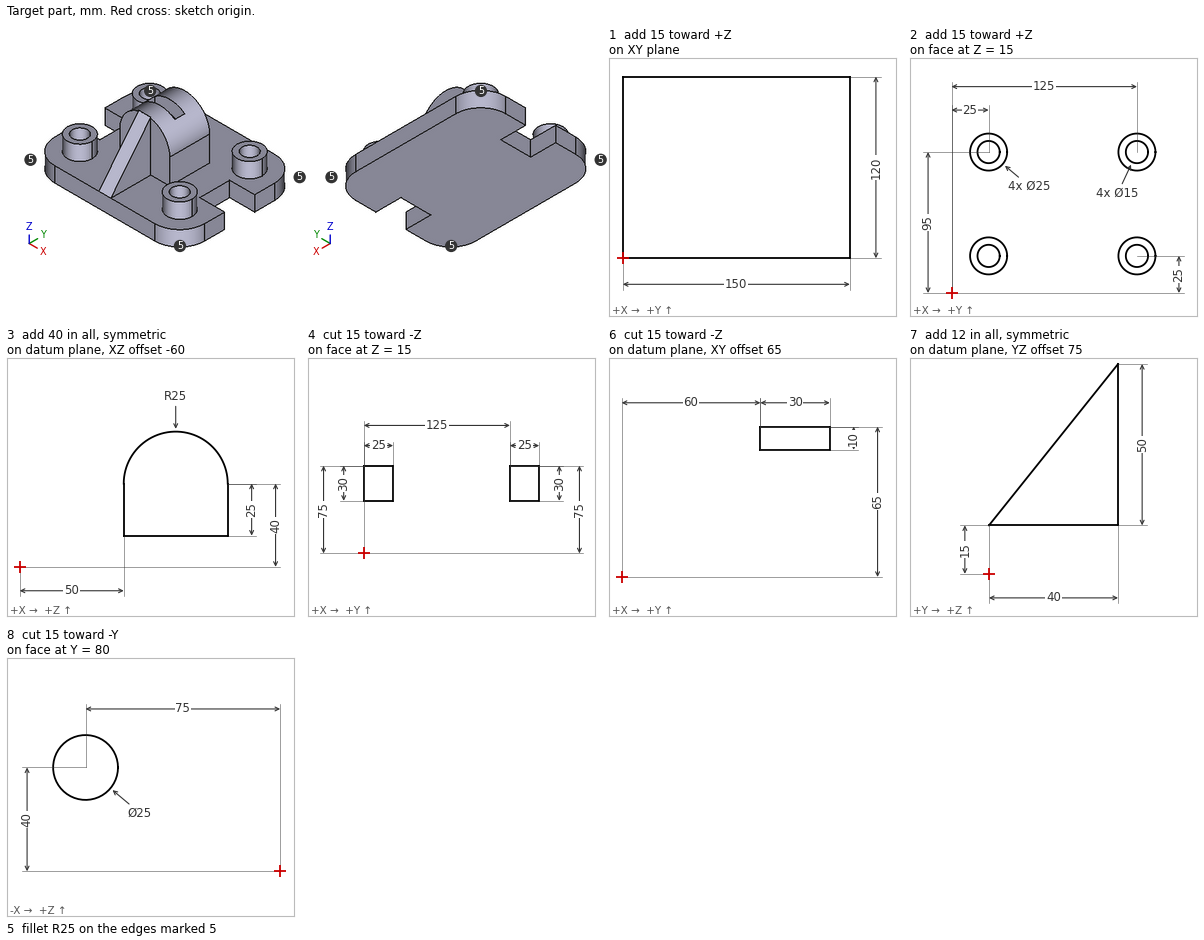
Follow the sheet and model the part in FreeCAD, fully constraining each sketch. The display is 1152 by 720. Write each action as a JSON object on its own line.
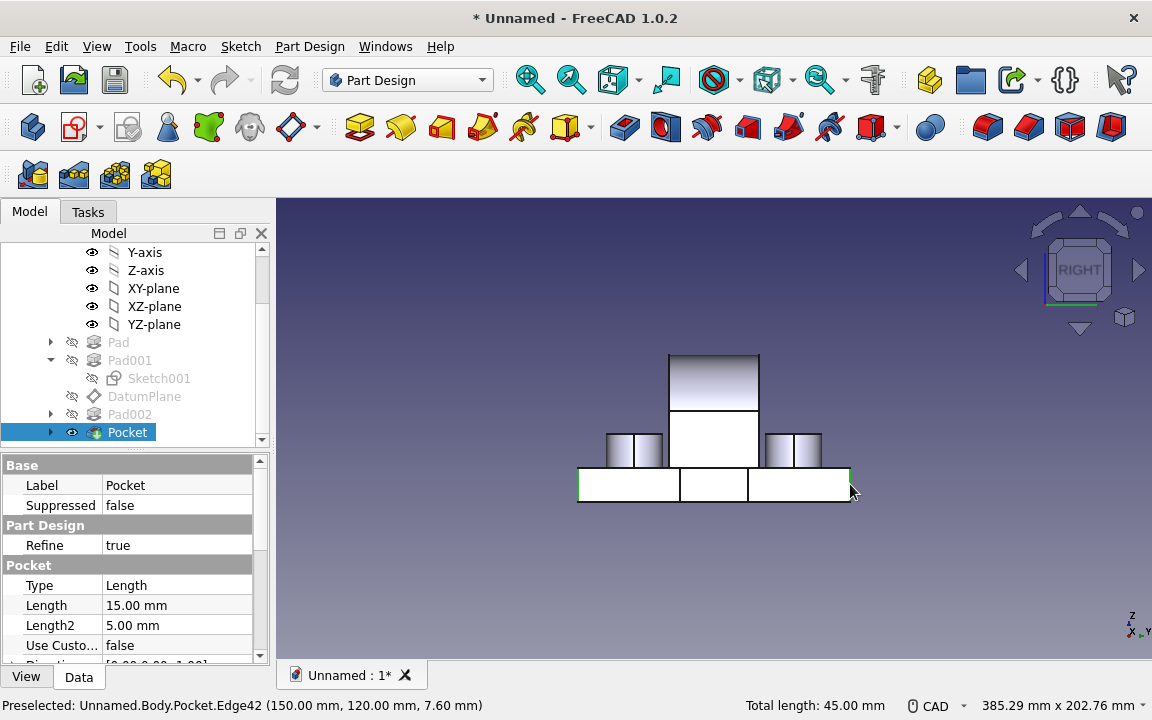
{"action": "key", "text": "5"}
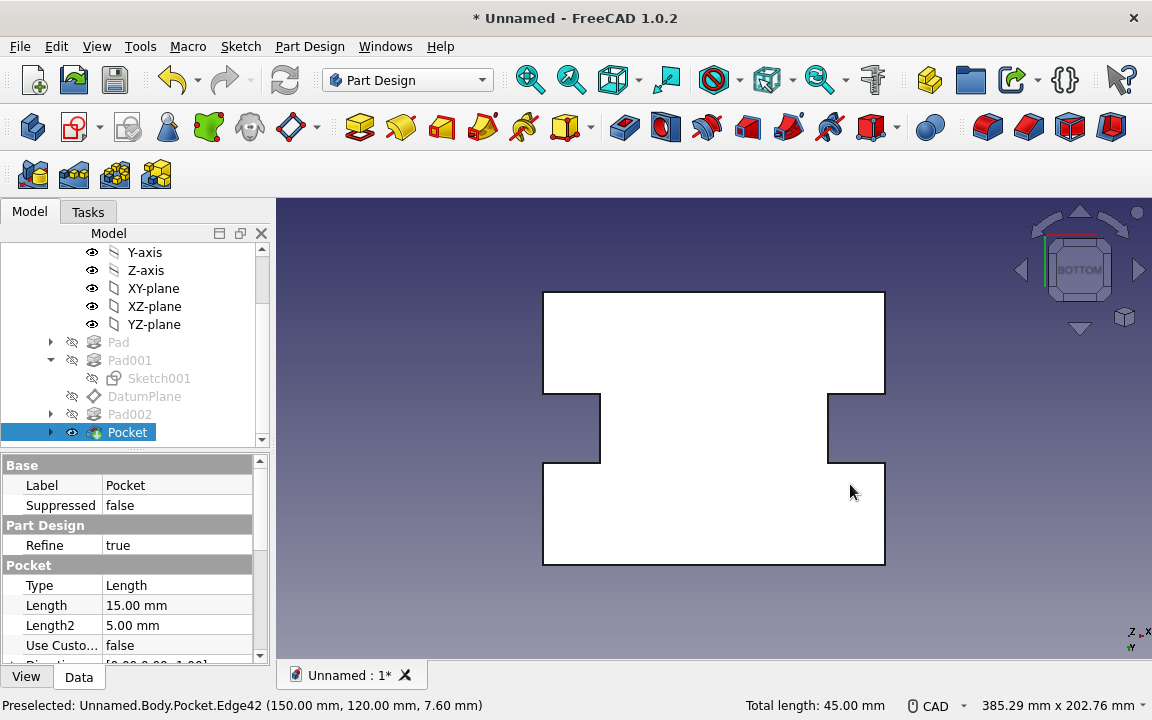
{"action": "key", "text": "4"}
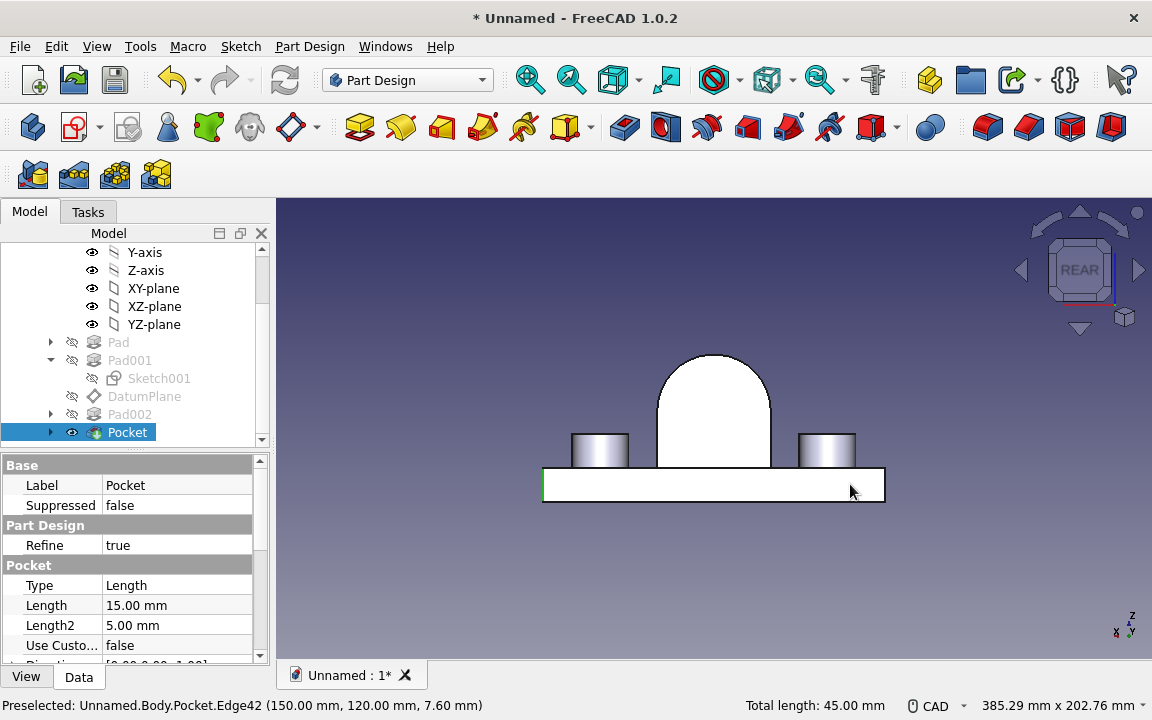
{"action": "left_click", "coordinate": [531, 80]}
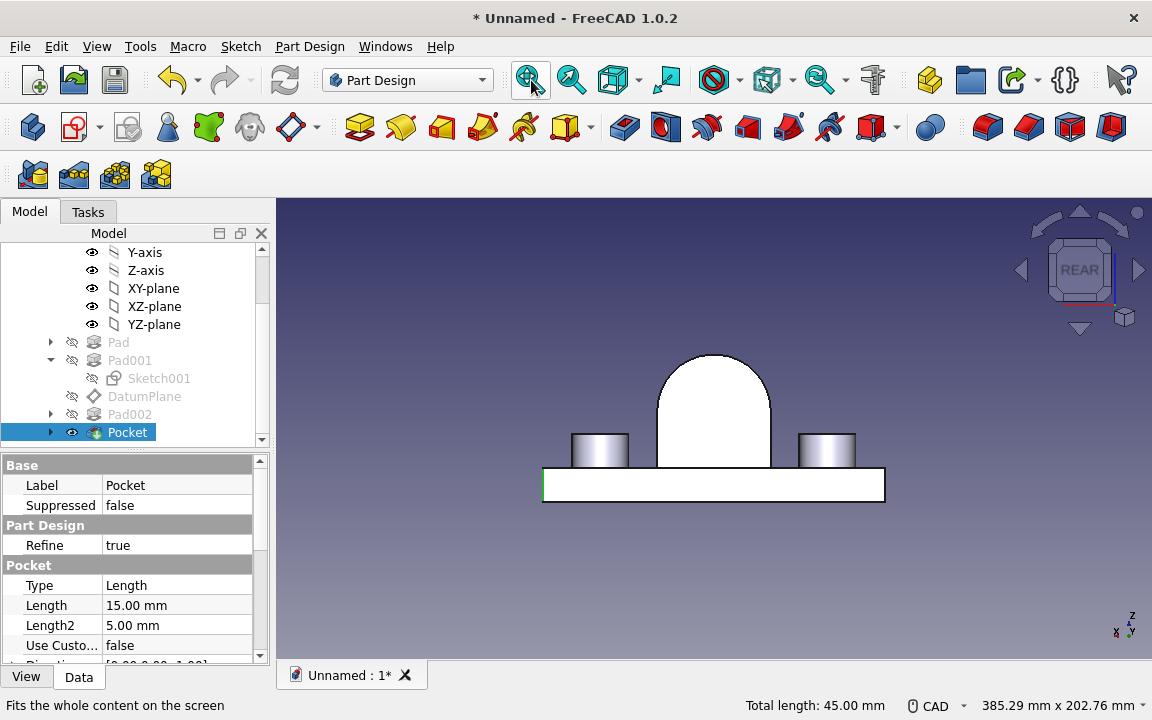
{"action": "left_click", "coordinate": [885, 484], "text": "ctrl"}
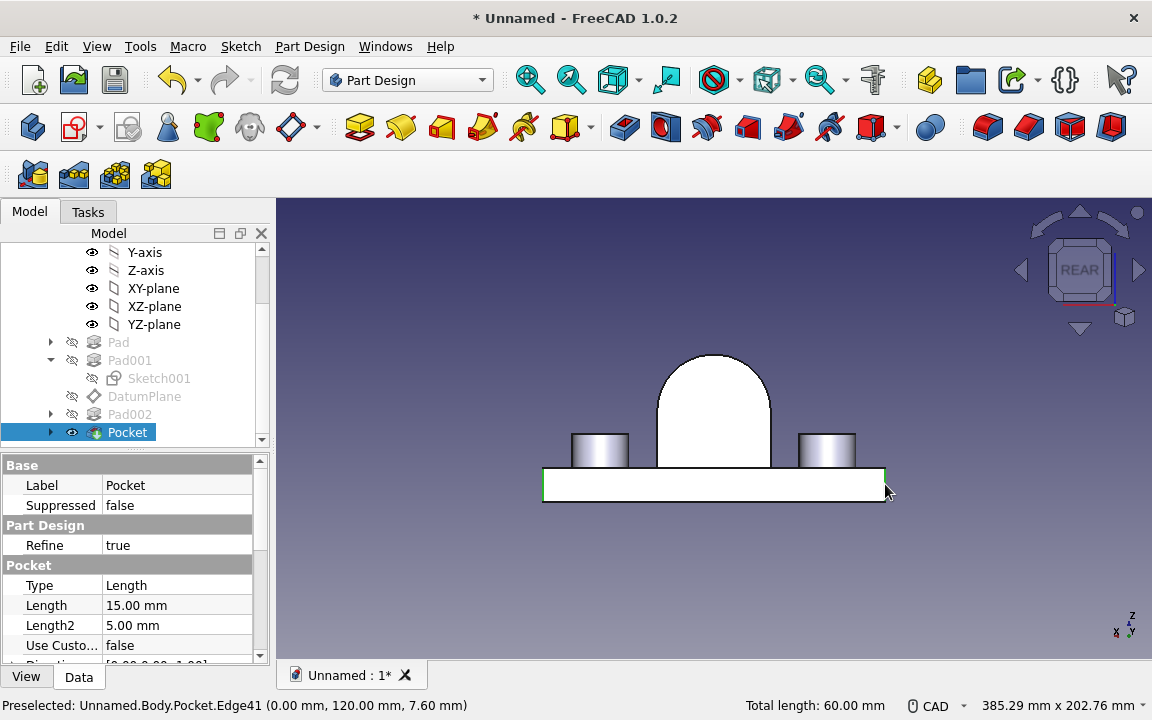
{"action": "left_click", "coordinate": [988, 128]}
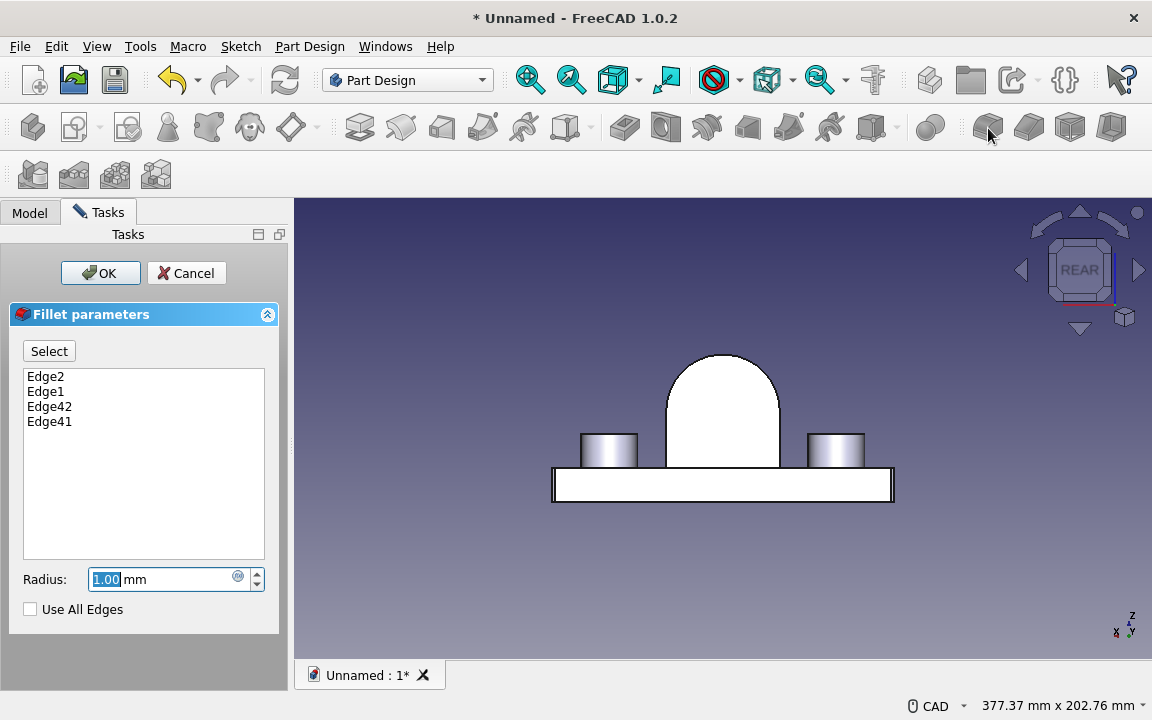
{"action": "type", "text": "25"}
{"action": "key", "text": "Tab"}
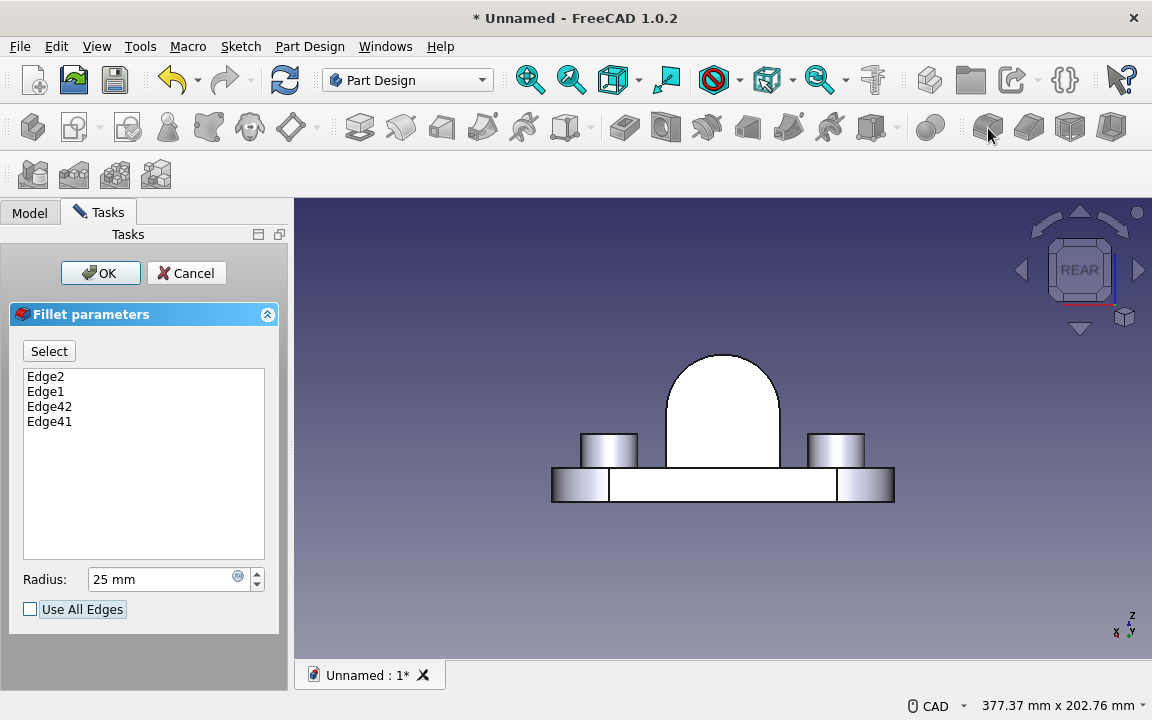
{"action": "left_click", "coordinate": [101, 273]}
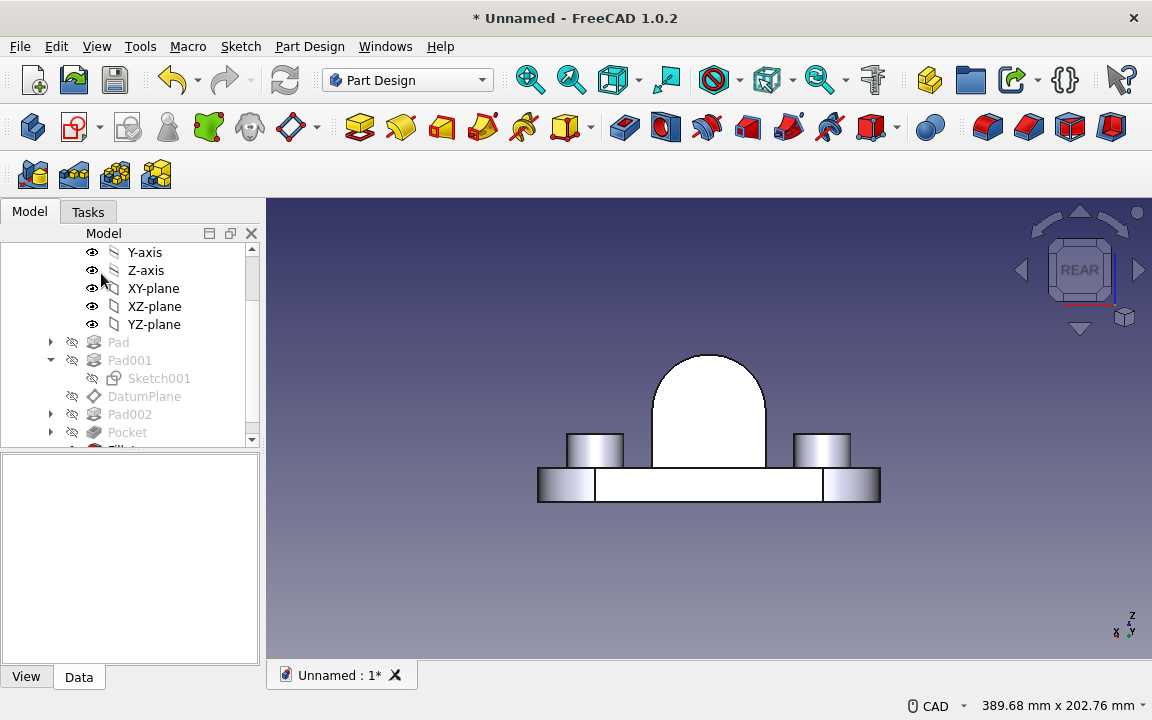
{"action": "left_click", "coordinate": [531, 80]}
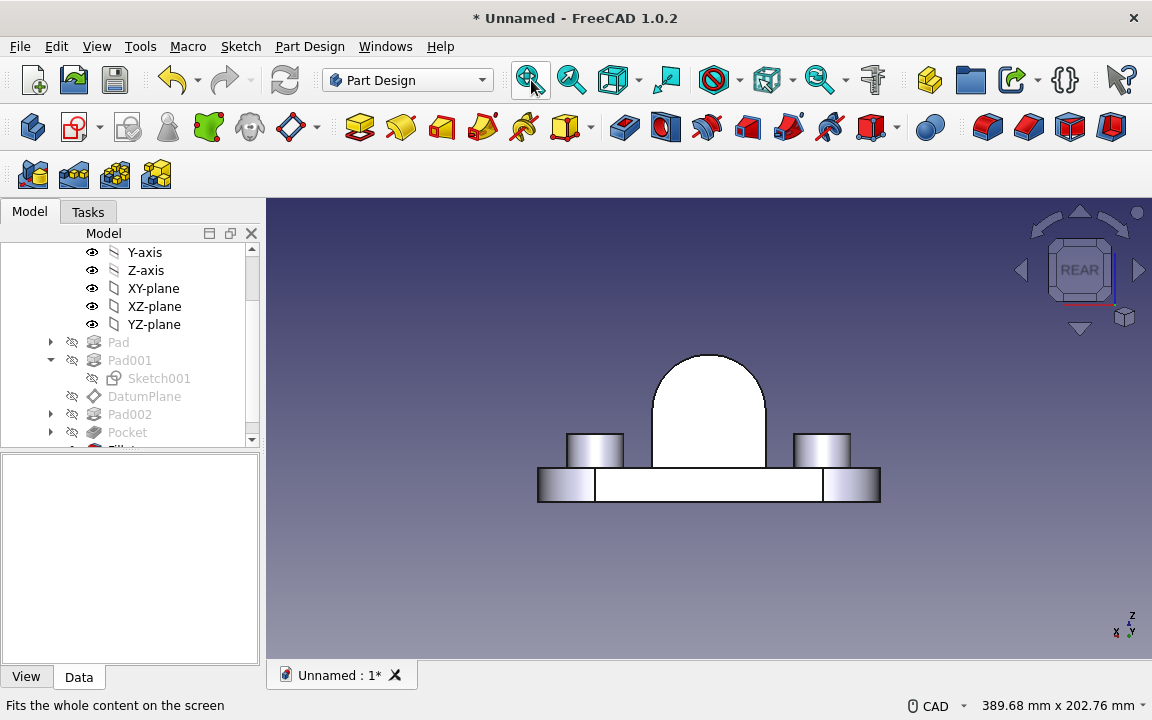
{"action": "scroll", "coordinate": [161, 338], "scroll_direction": "down", "scroll_amount": 3}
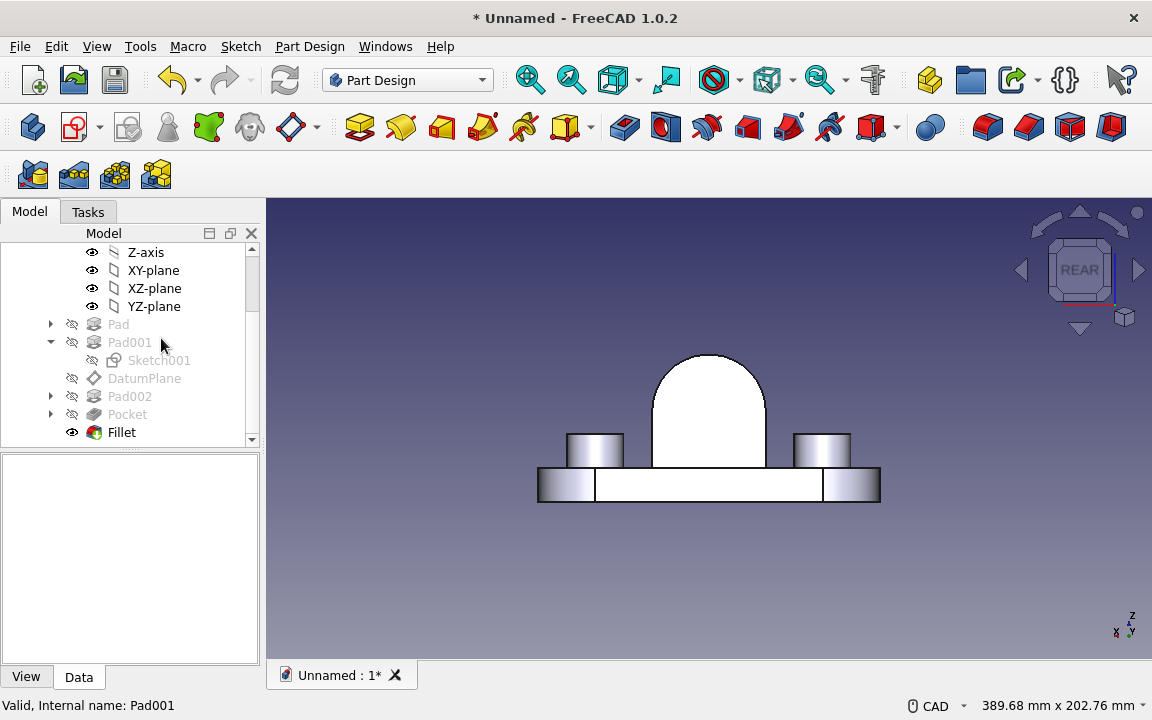
{"action": "scroll", "coordinate": [161, 338], "scroll_direction": "up", "scroll_amount": 15}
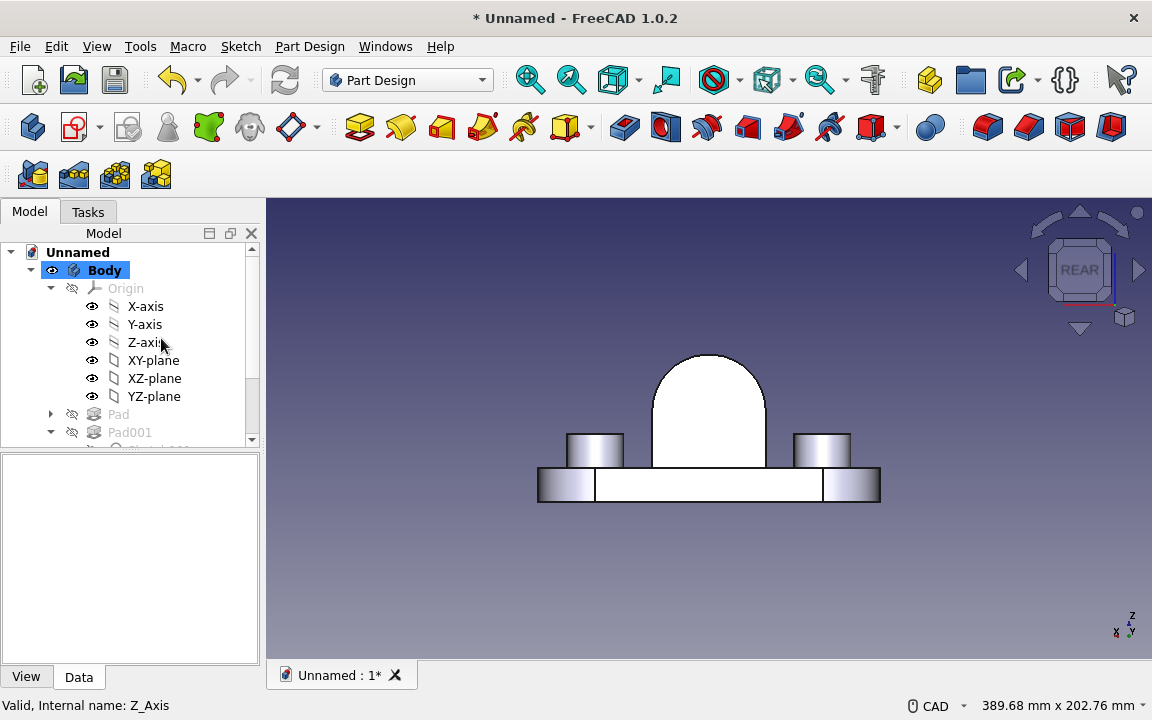
{"action": "left_click", "coordinate": [137, 360]}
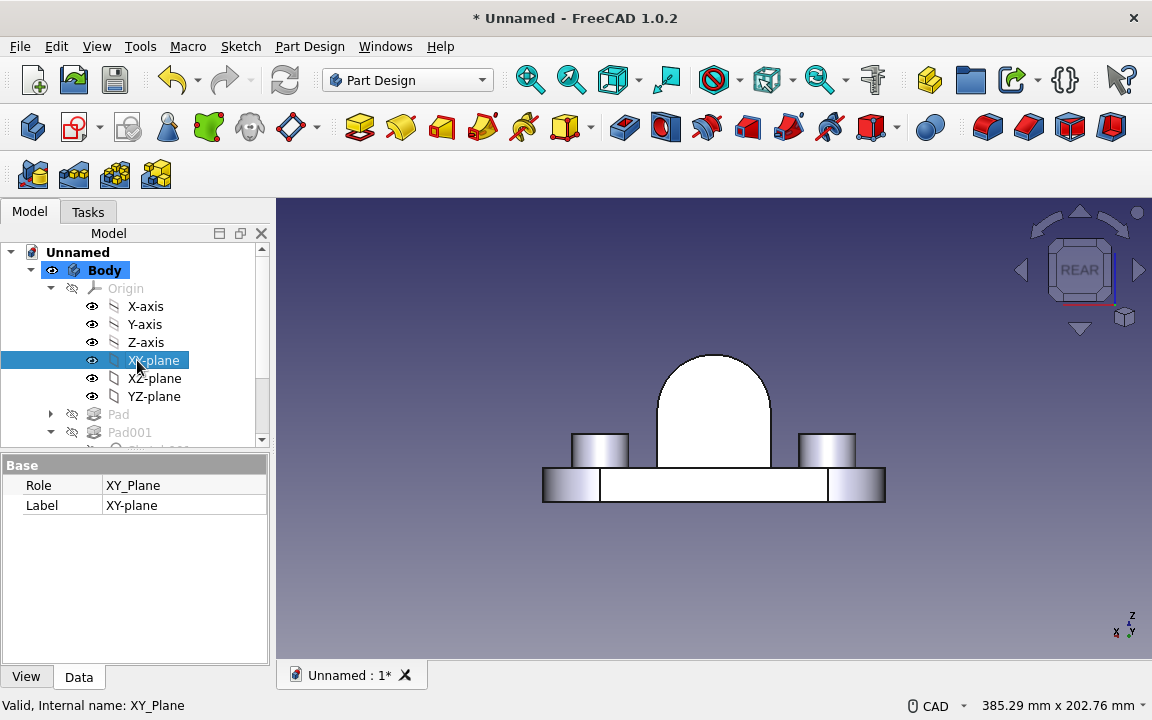
{"action": "left_click", "coordinate": [290, 128]}